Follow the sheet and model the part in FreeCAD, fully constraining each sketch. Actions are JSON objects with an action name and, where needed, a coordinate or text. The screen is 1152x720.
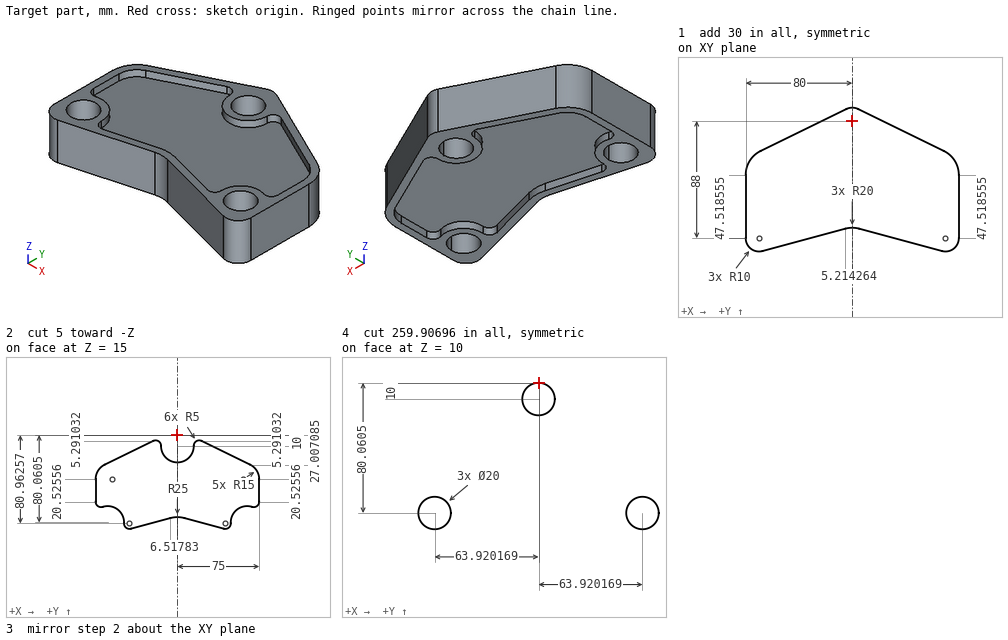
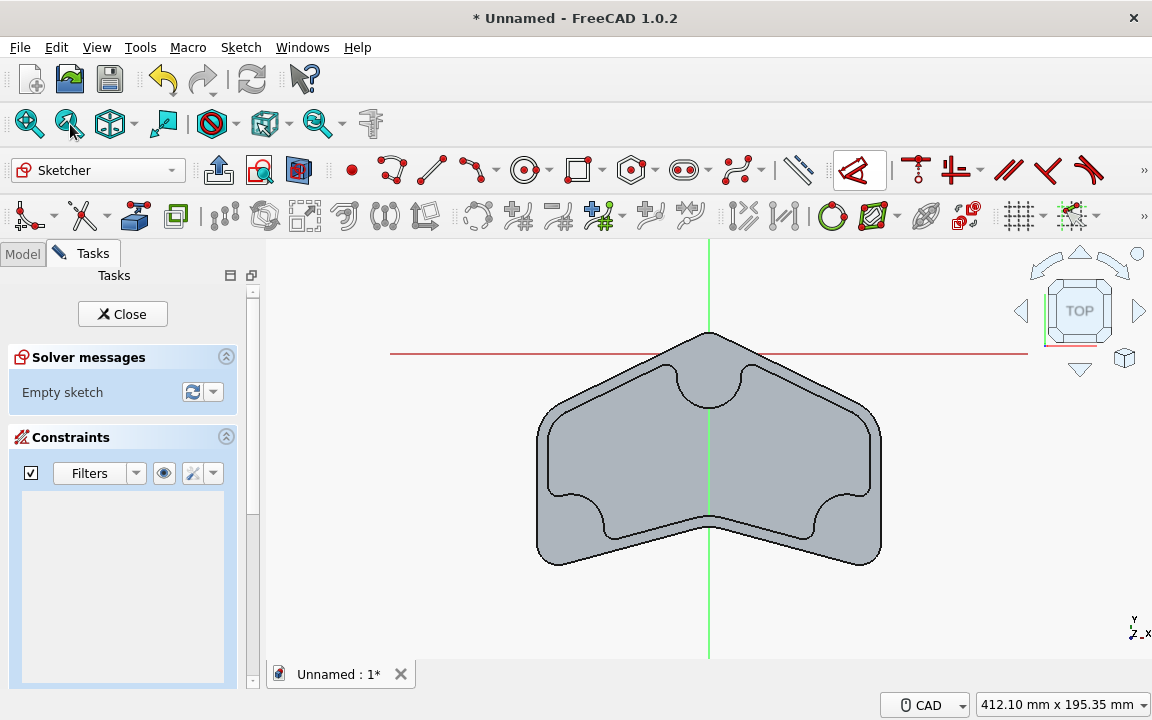
{"action": "left_click", "coordinate": [526, 170]}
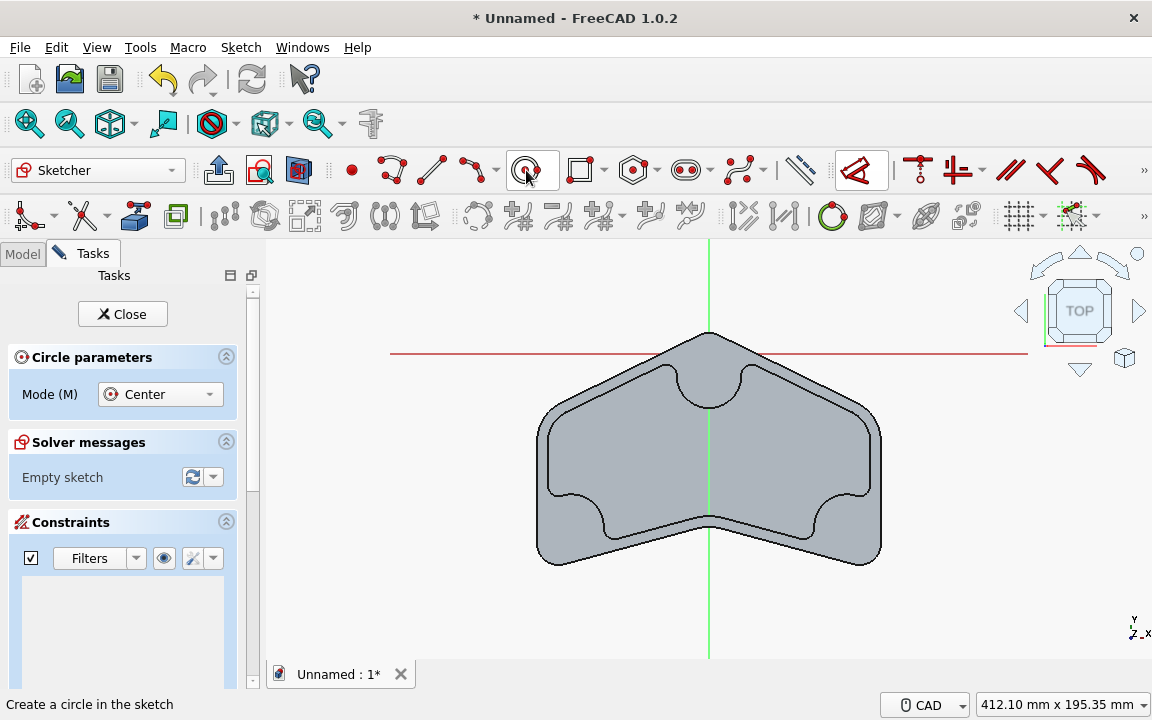
{"action": "left_click", "coordinate": [572, 527]}
{"action": "left_click", "coordinate": [587, 511]}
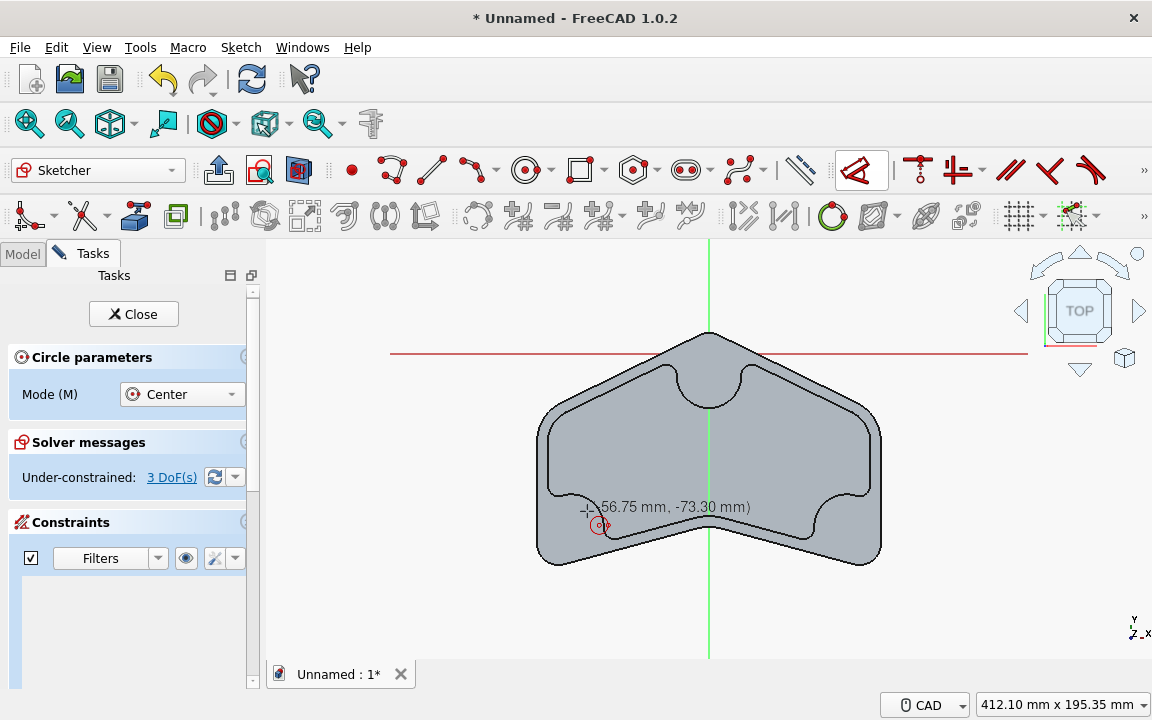
{"action": "left_click", "coordinate": [709, 376]}
{"action": "left_click", "coordinate": [724, 391]}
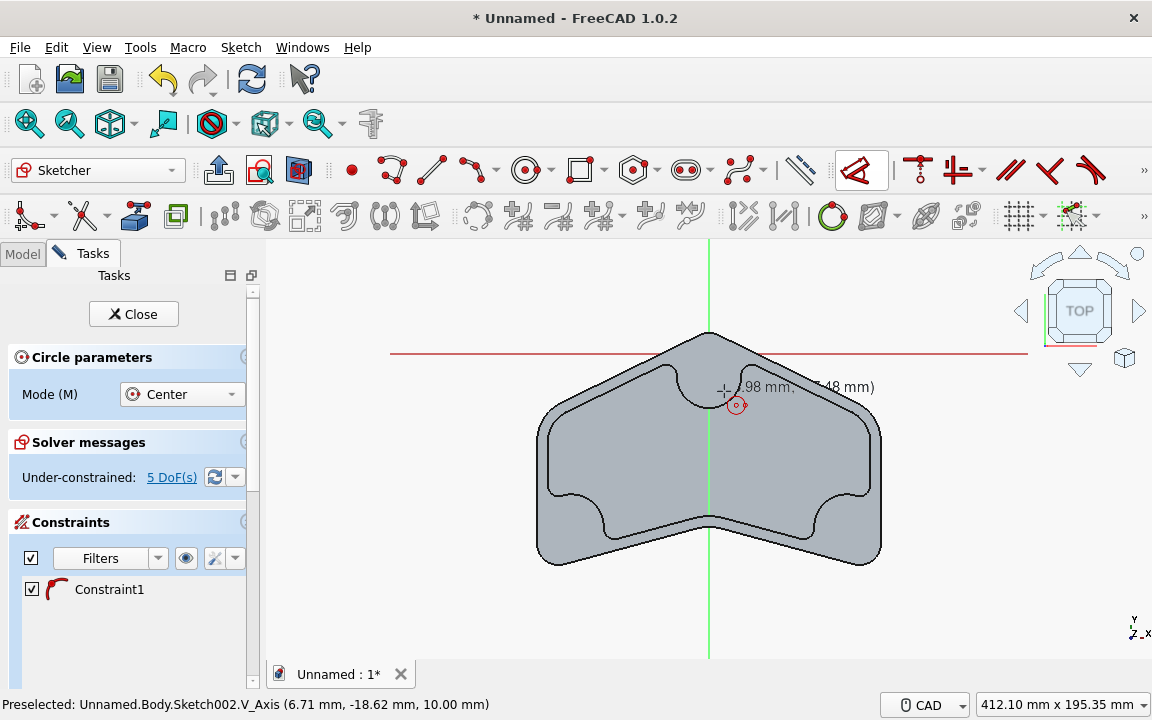
{"action": "left_click", "coordinate": [846, 527]}
{"action": "left_click", "coordinate": [862, 511]}
{"action": "key", "text": "Escape"}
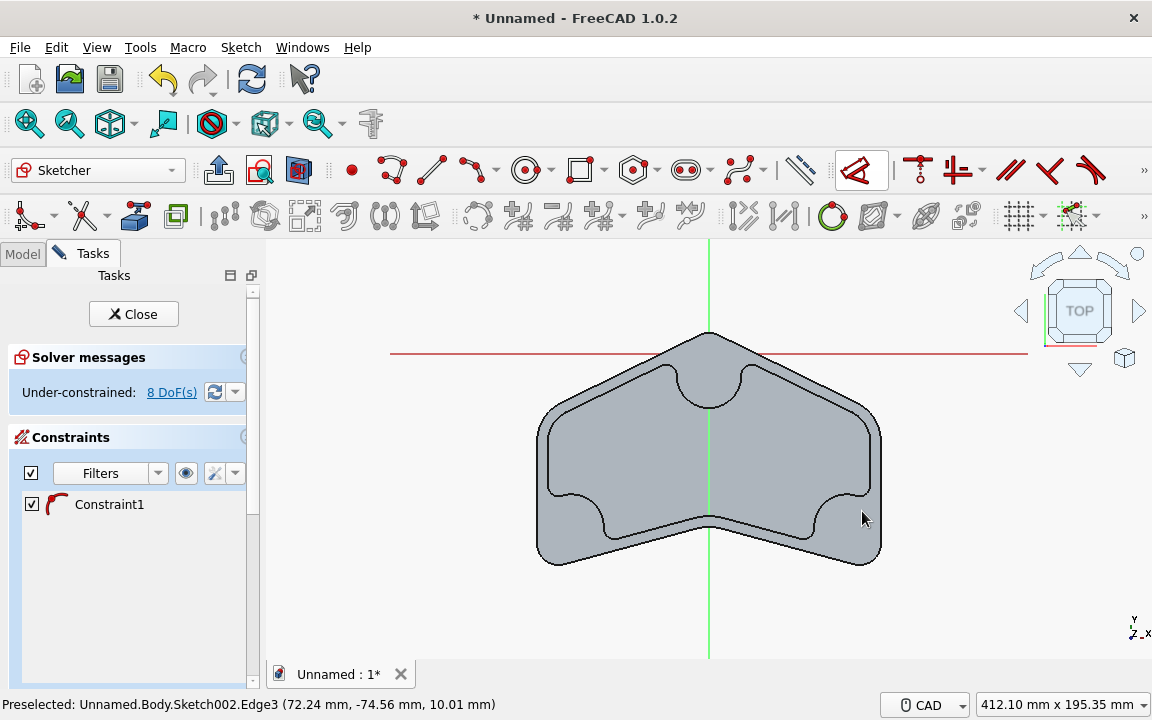
{"action": "left_click", "coordinate": [587, 512]}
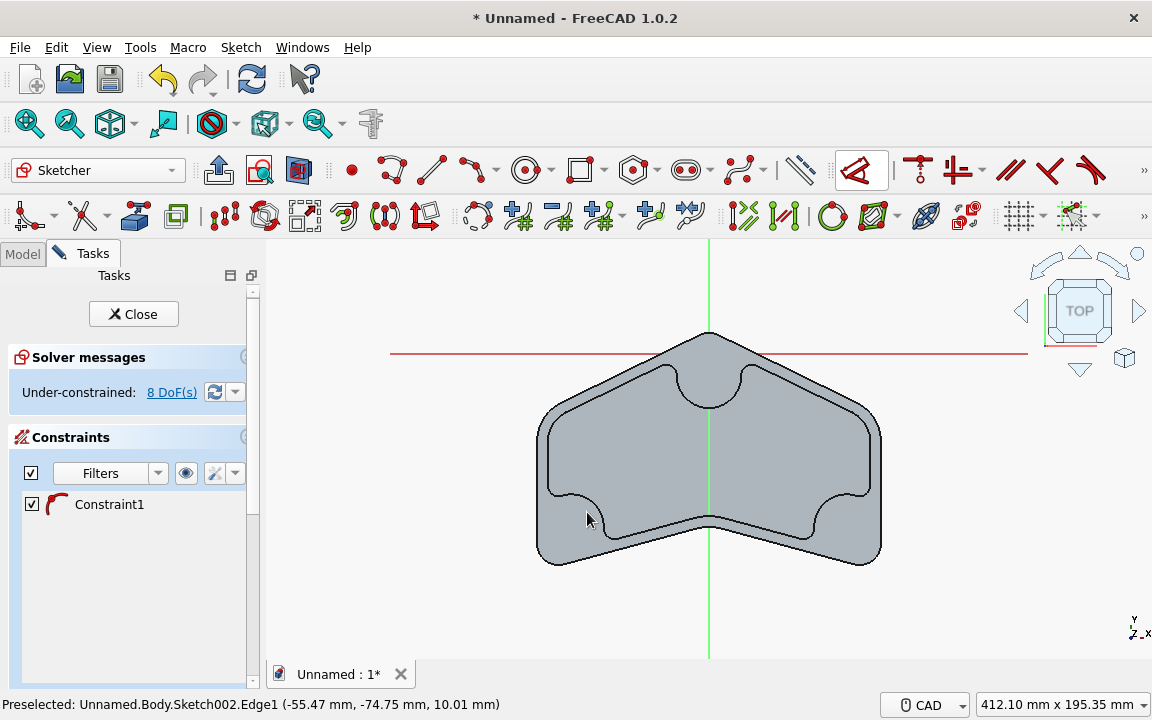
{"action": "left_click", "coordinate": [694, 392]}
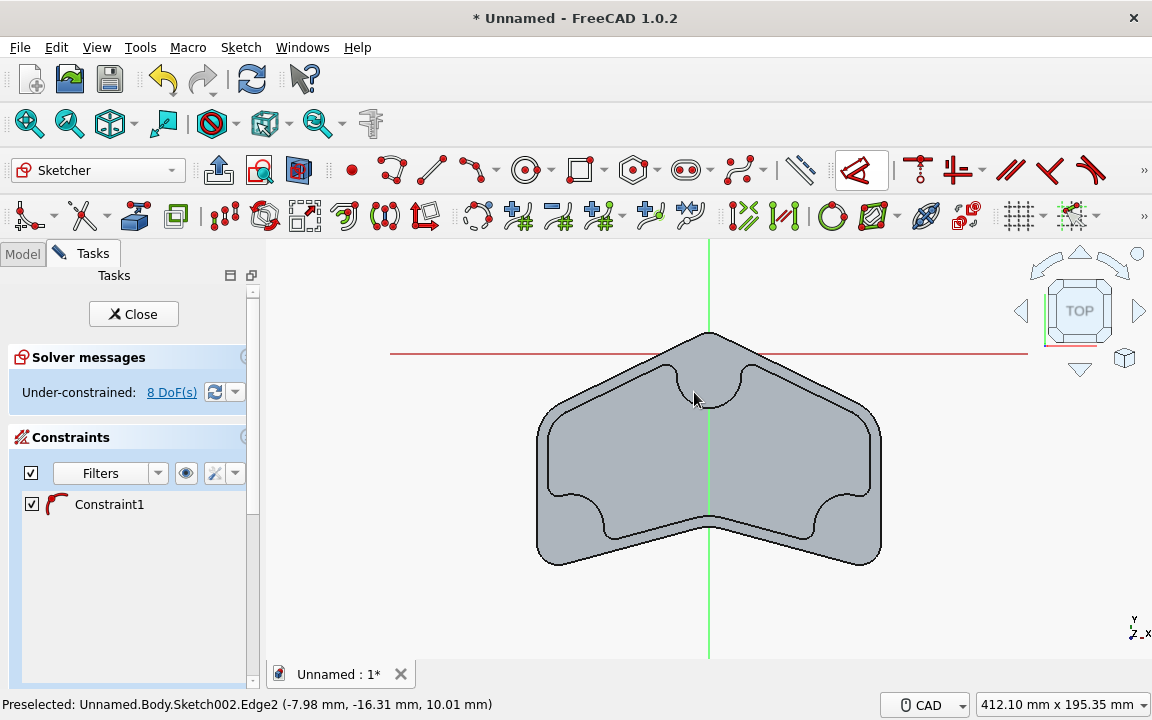
{"action": "left_click", "coordinate": [862, 512]}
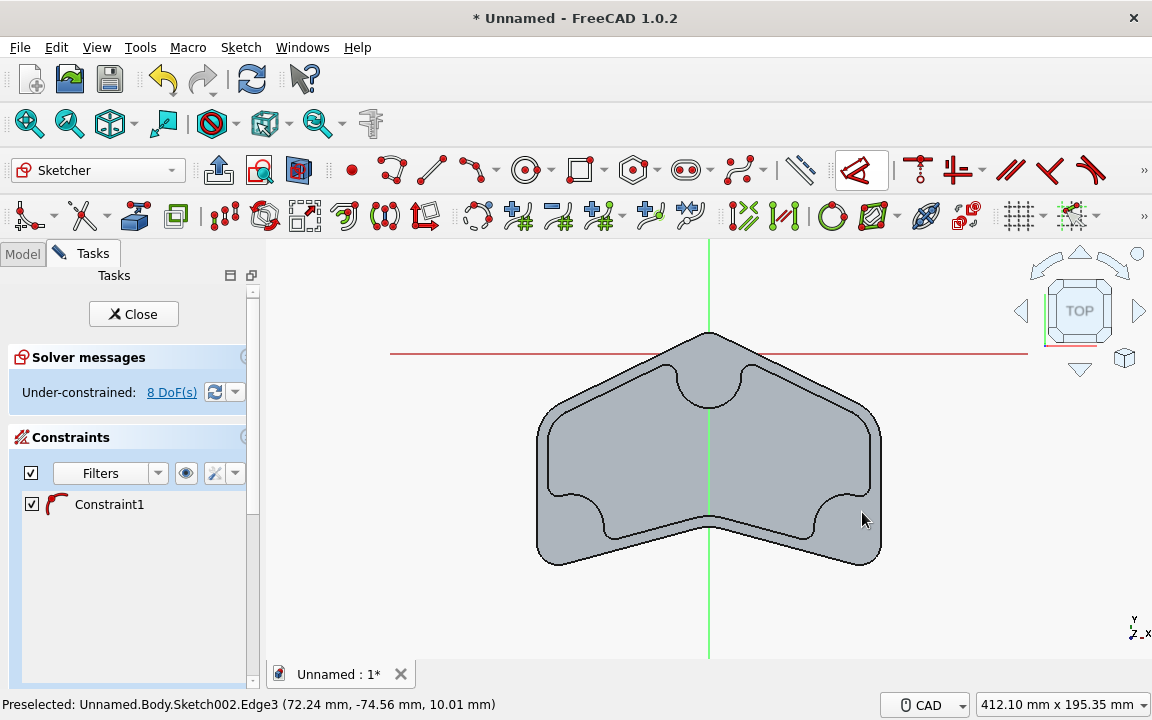
{"action": "key", "text": "e"}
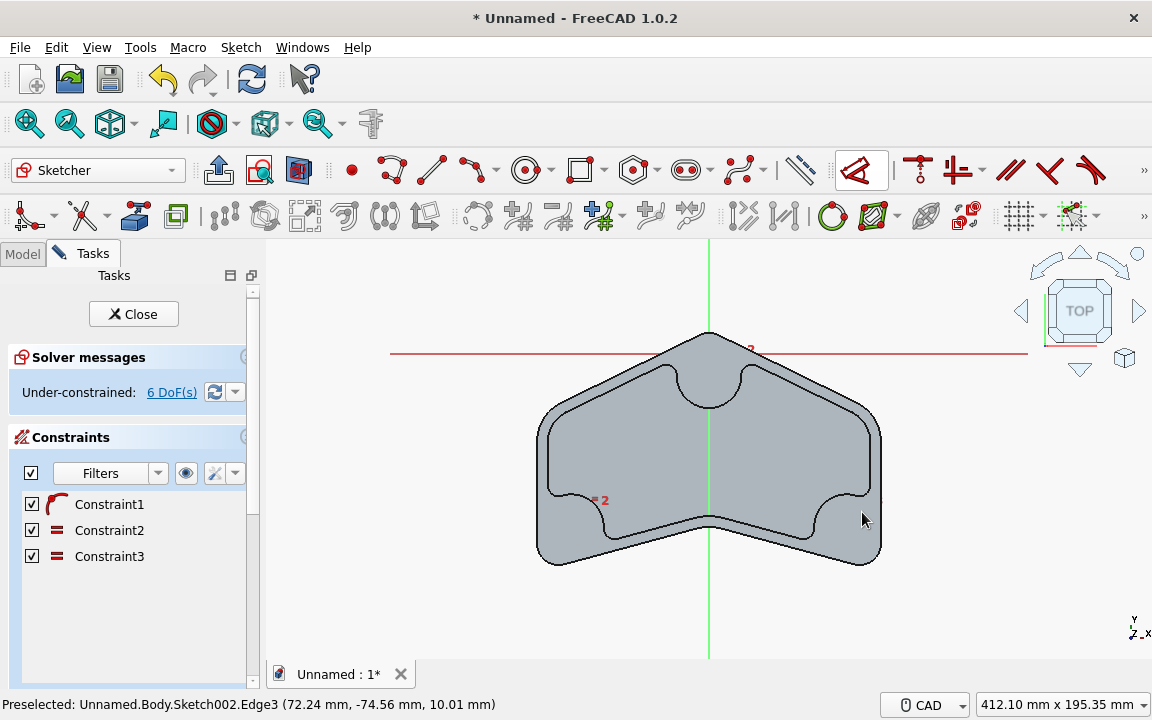
{"action": "left_click", "coordinate": [572, 528]}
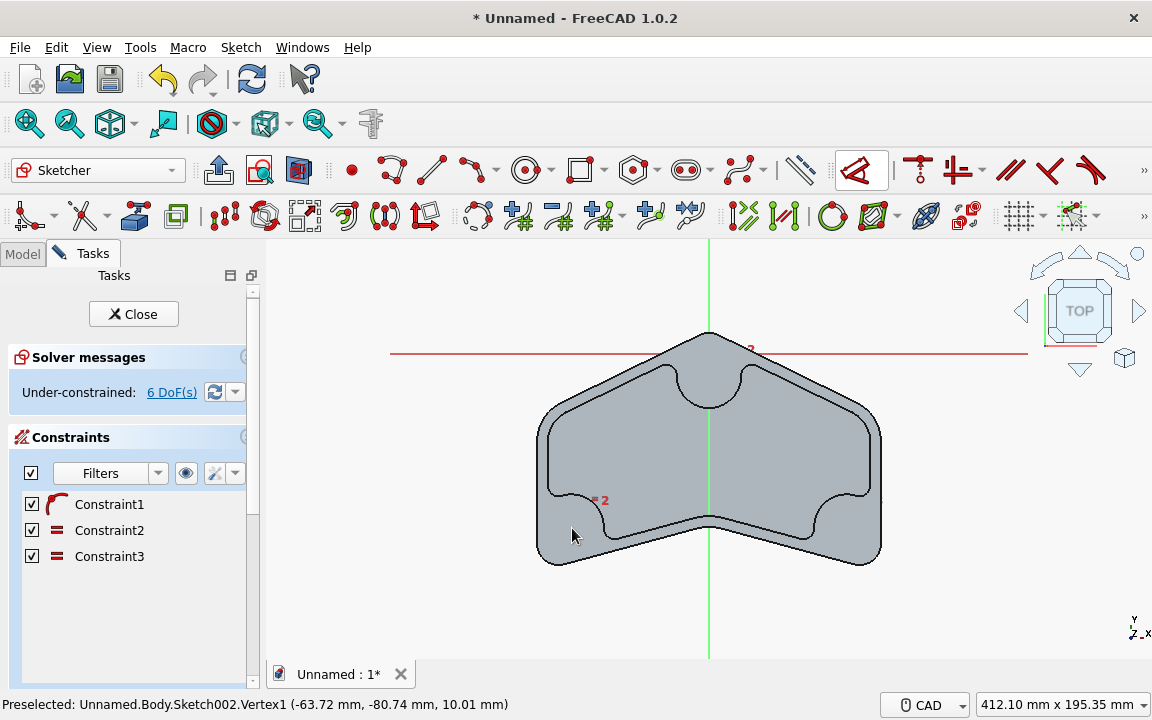
{"action": "left_click", "coordinate": [846, 528]}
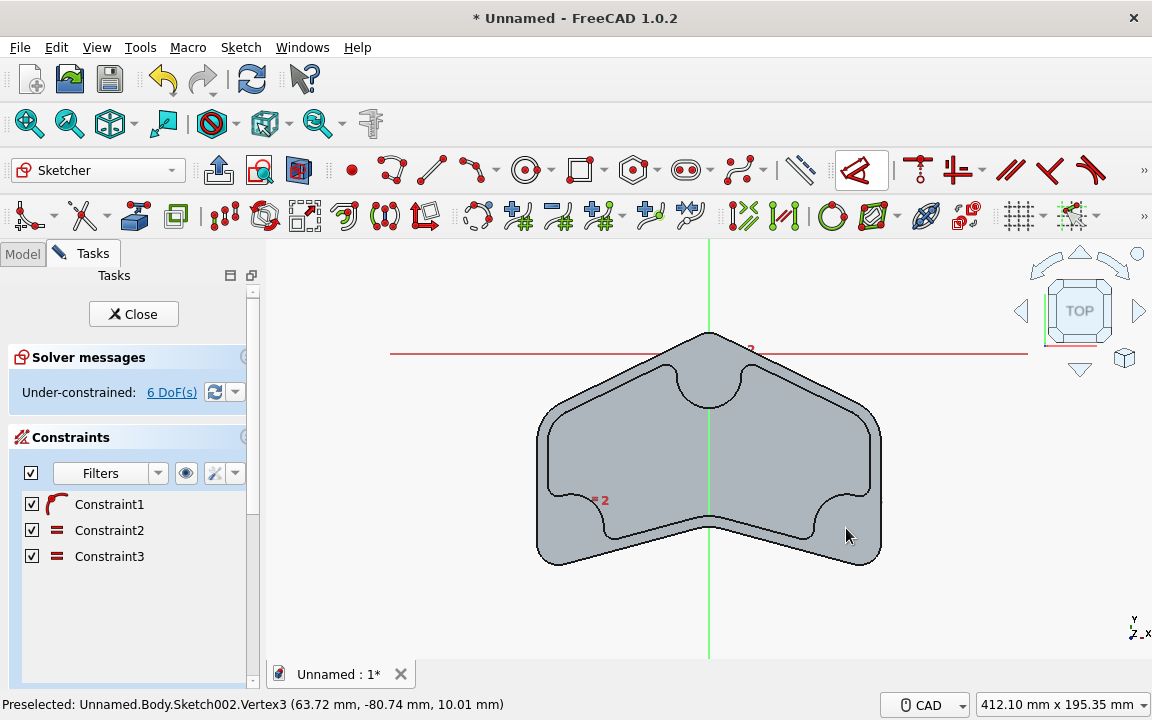
{"action": "left_click", "coordinate": [984, 170]}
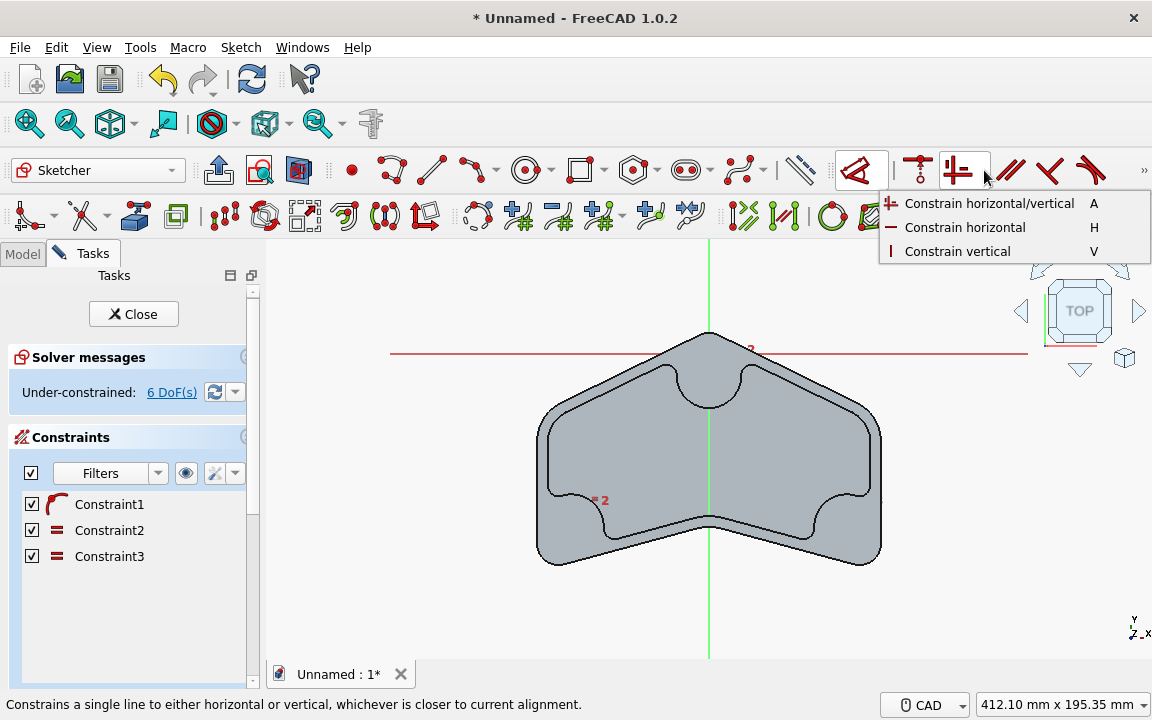
{"action": "left_click", "coordinate": [1015, 227]}